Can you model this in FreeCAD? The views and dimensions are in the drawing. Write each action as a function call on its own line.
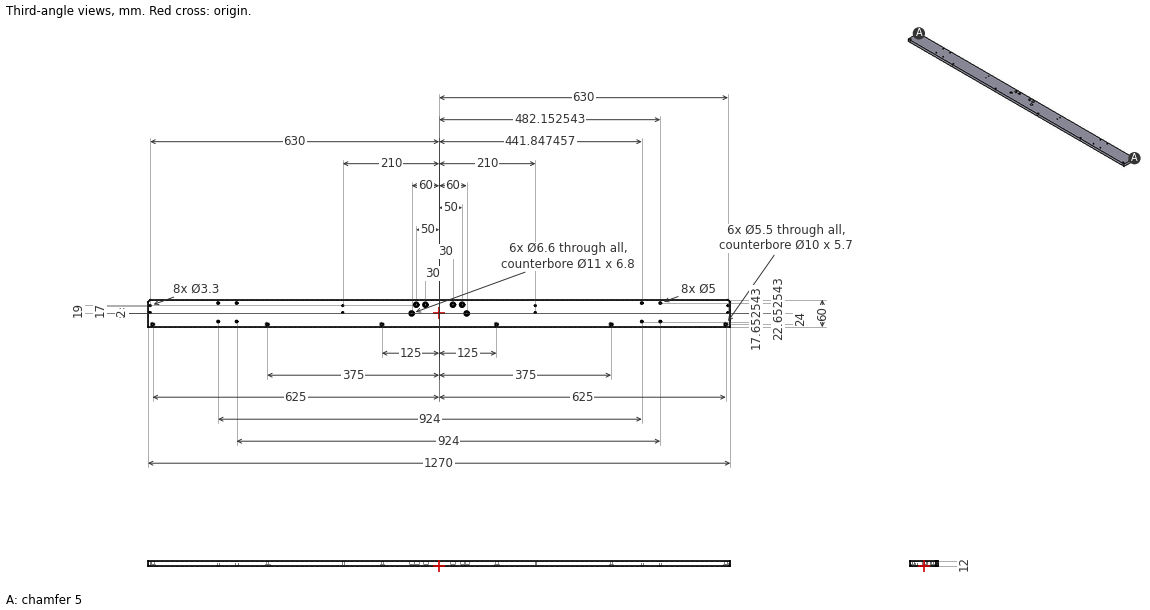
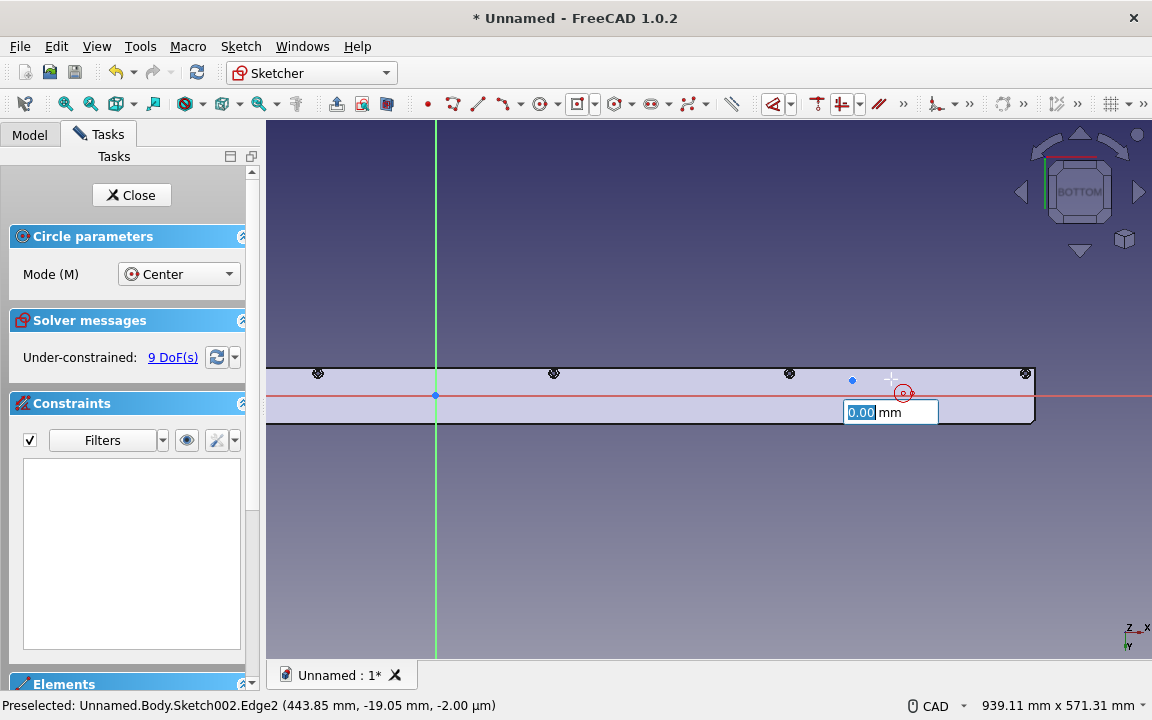
scroll(892, 378, up, 10)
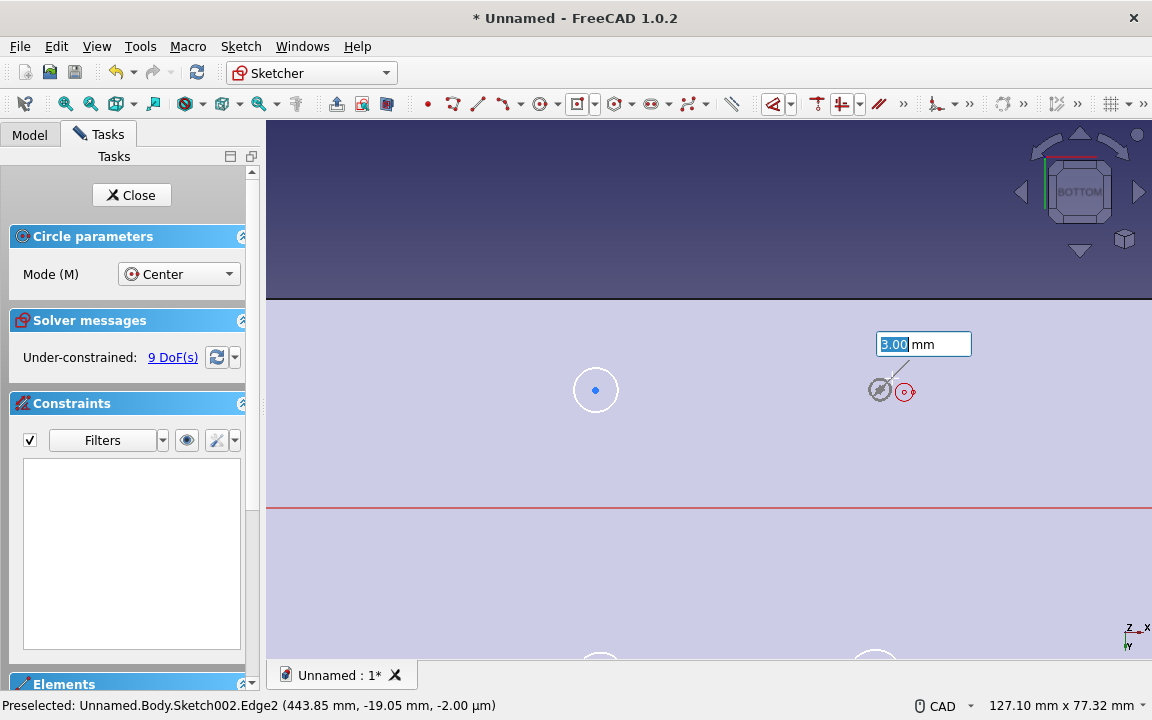
click(891, 373)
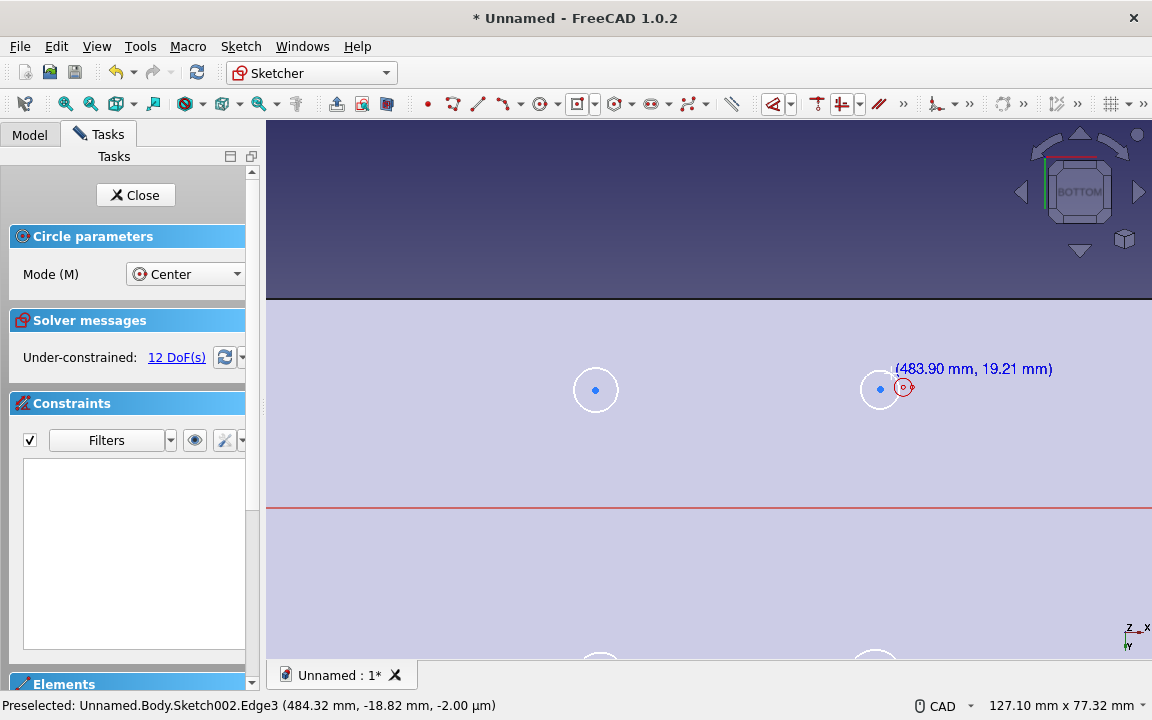
scroll(891, 379, down, 13)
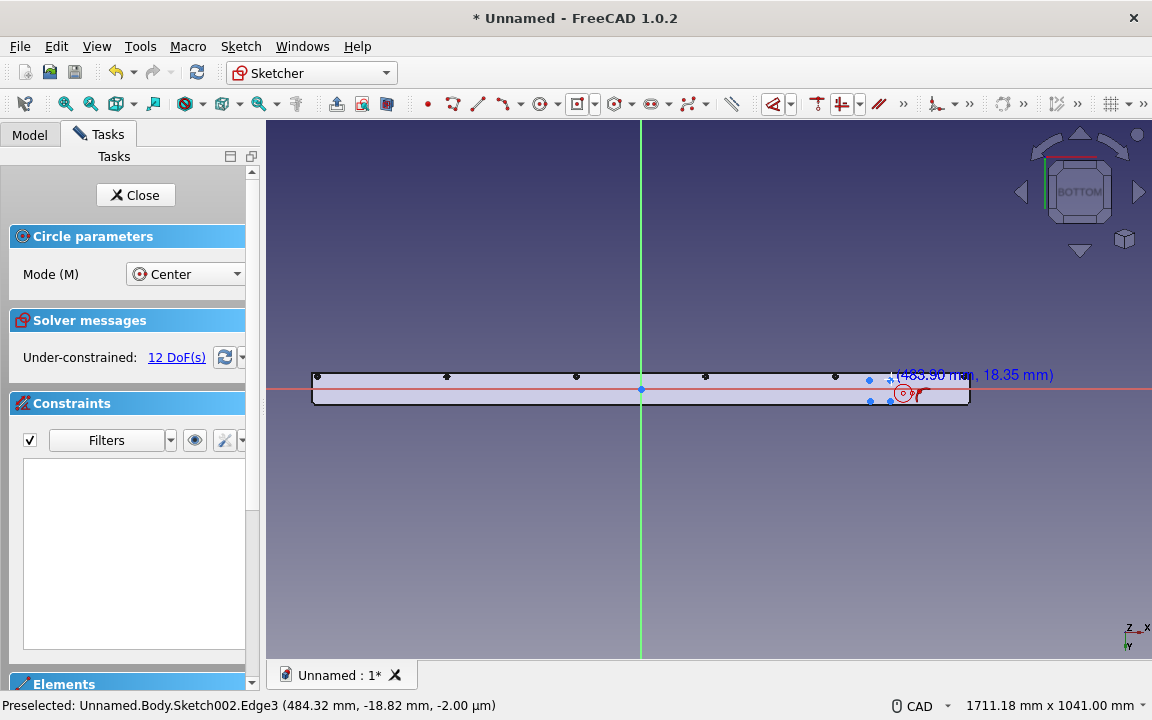
scroll(391, 380, up, 15)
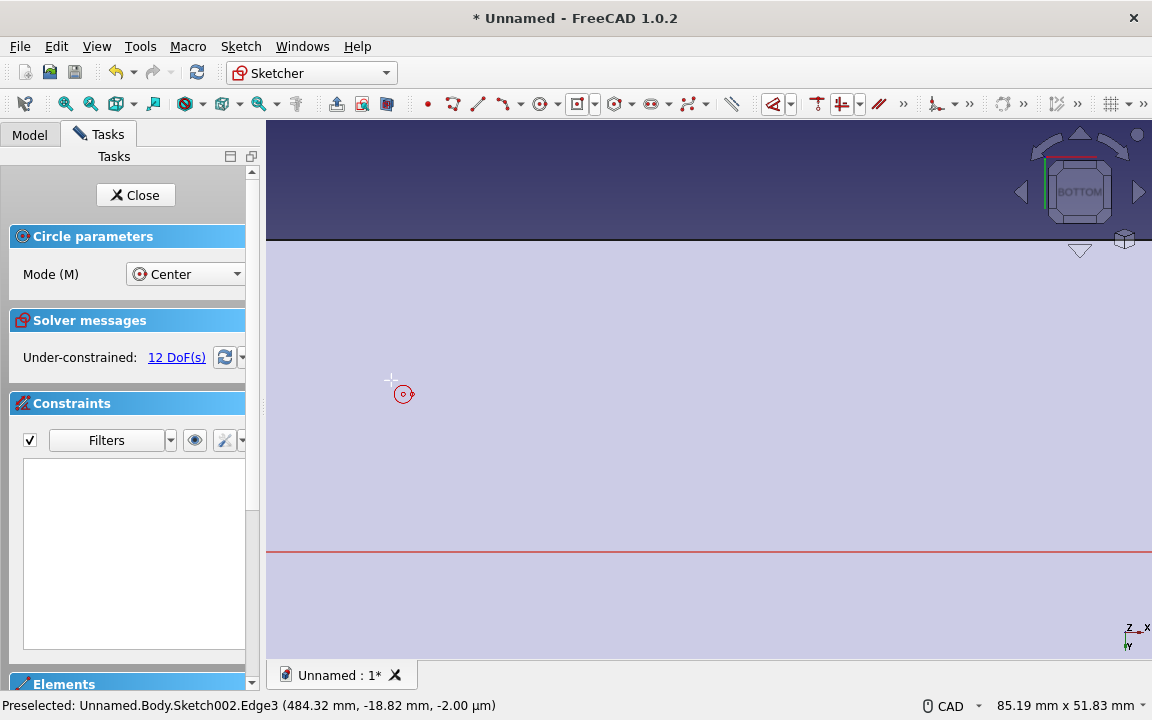
scroll(391, 380, down, 15)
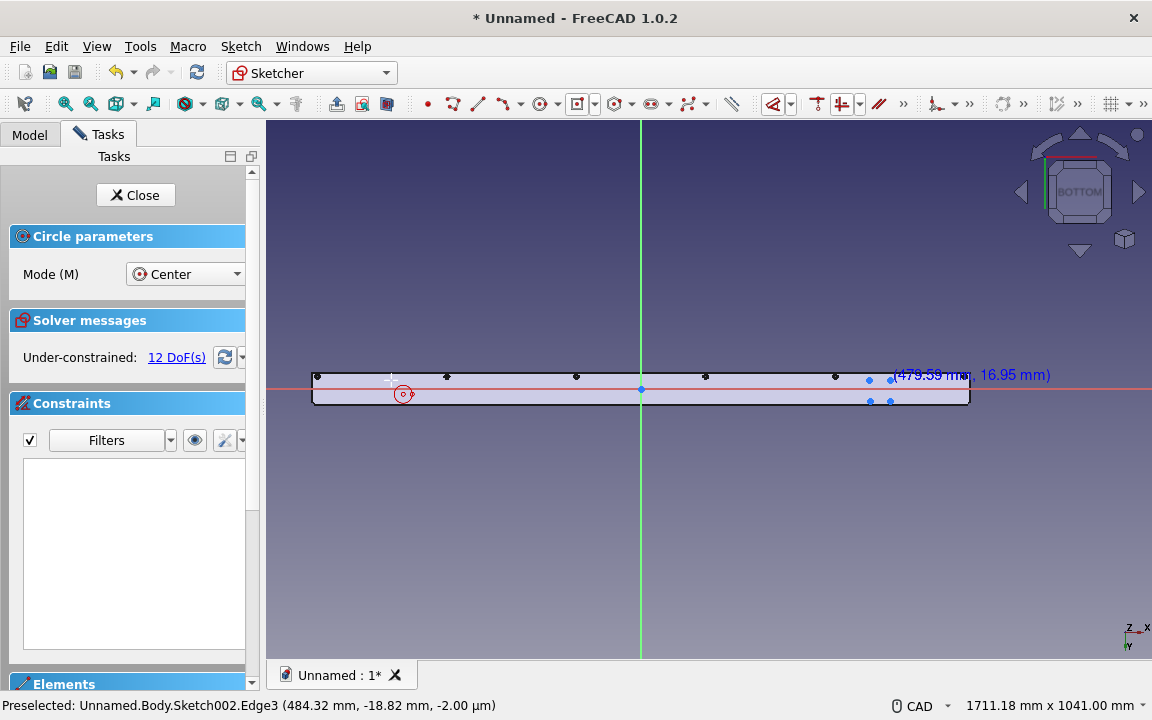
scroll(391, 380, up, 3)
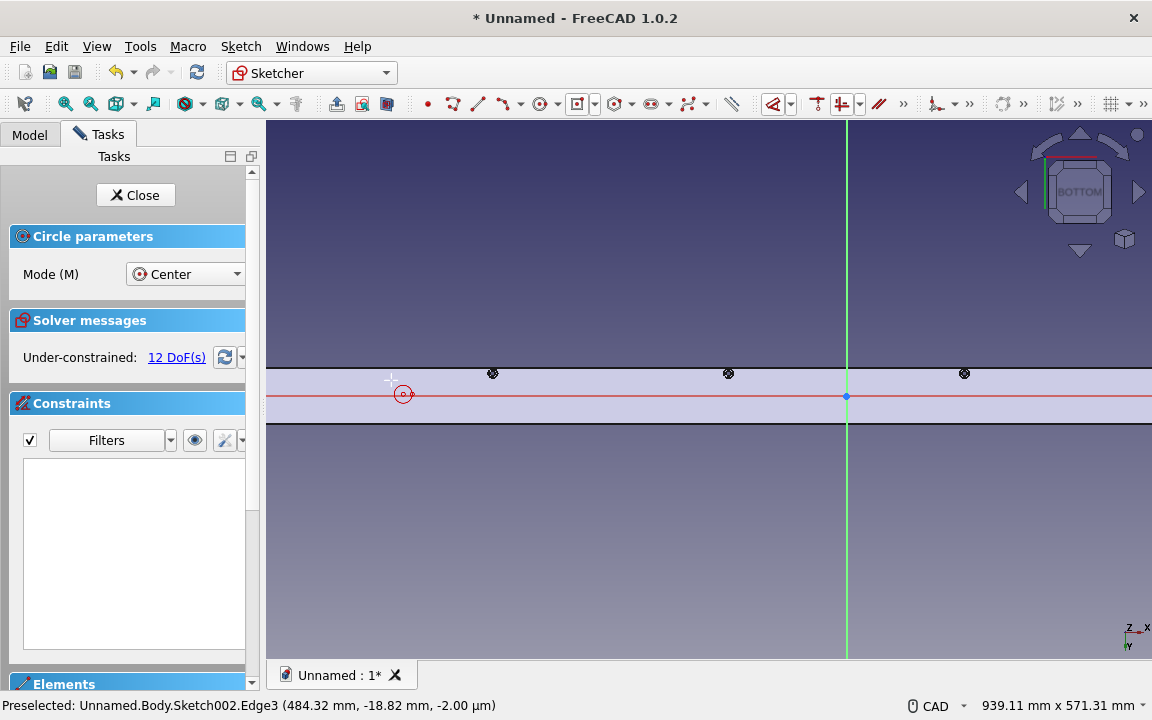
click(392, 379)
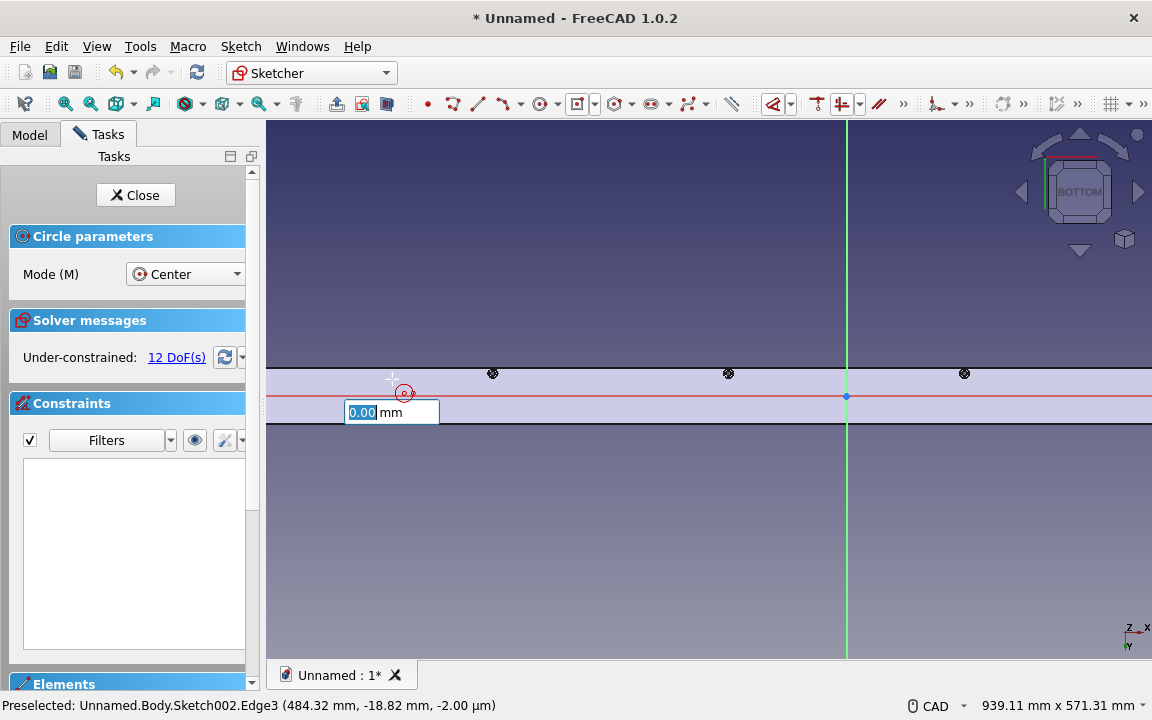
scroll(393, 378, up, 10)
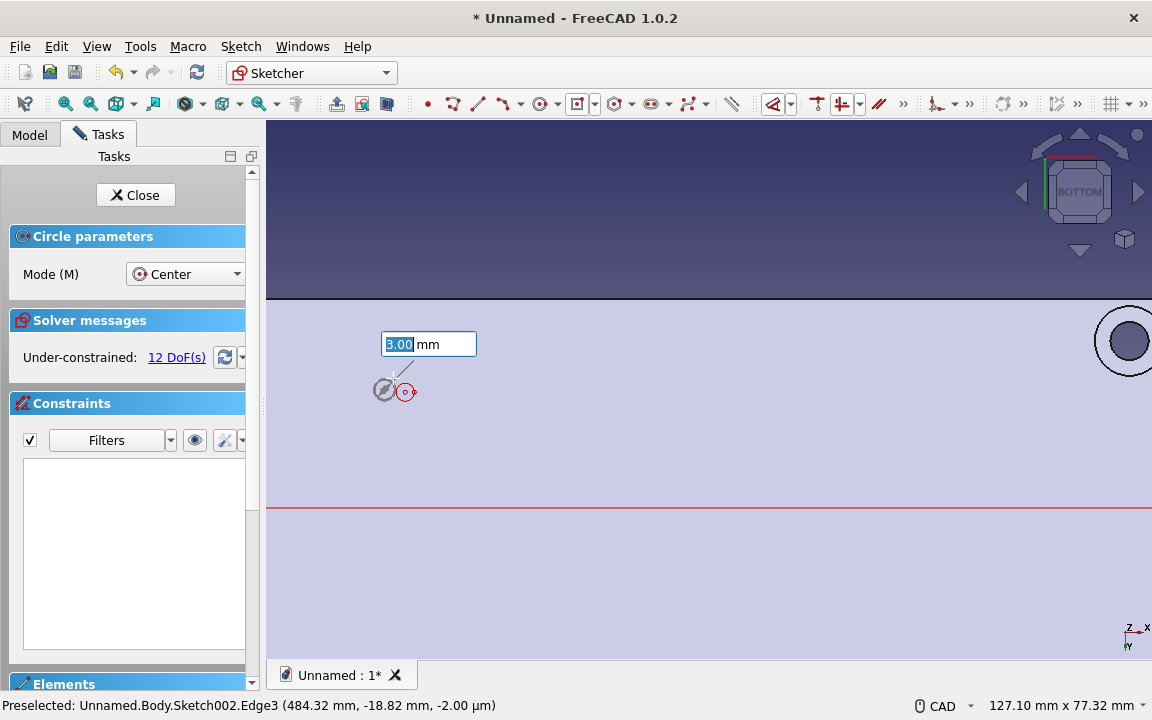
click(395, 373)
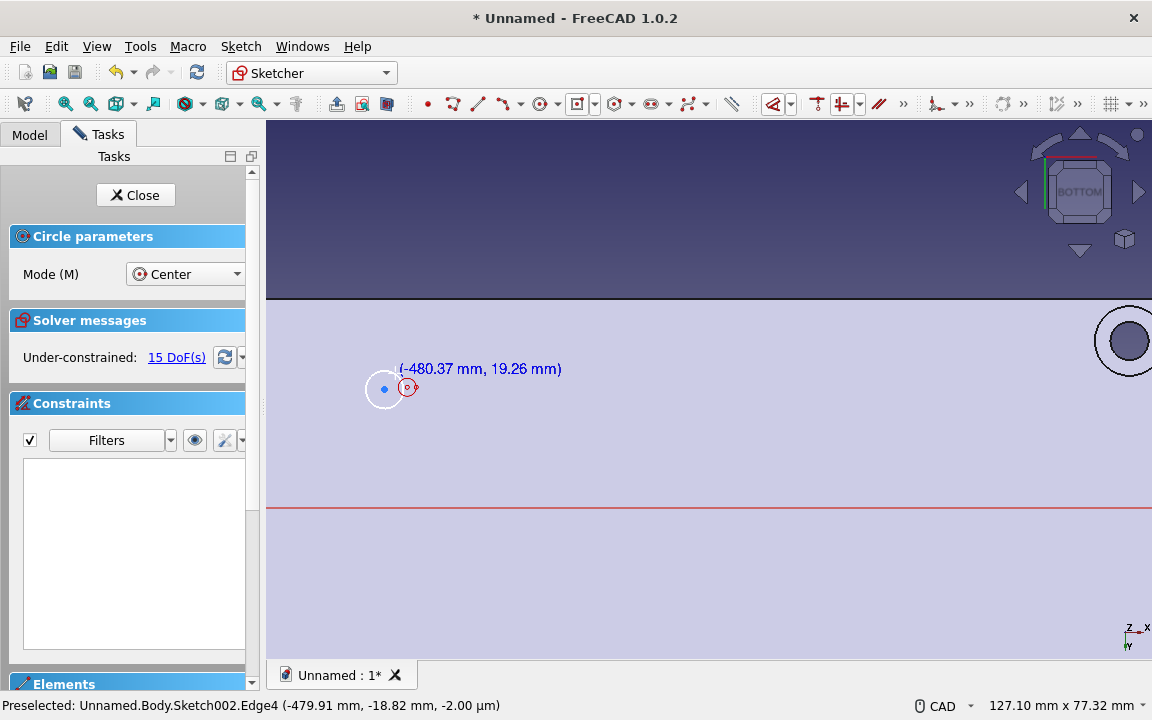
scroll(664, 385, up, 2)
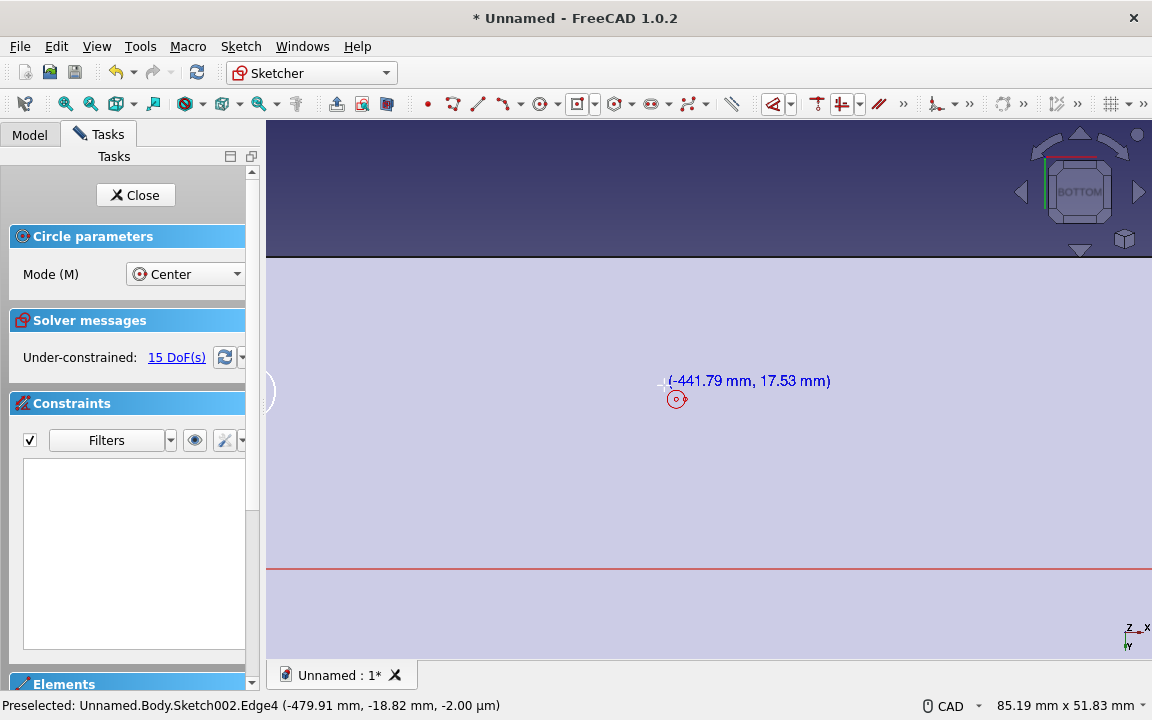
scroll(399, 379, down, 15)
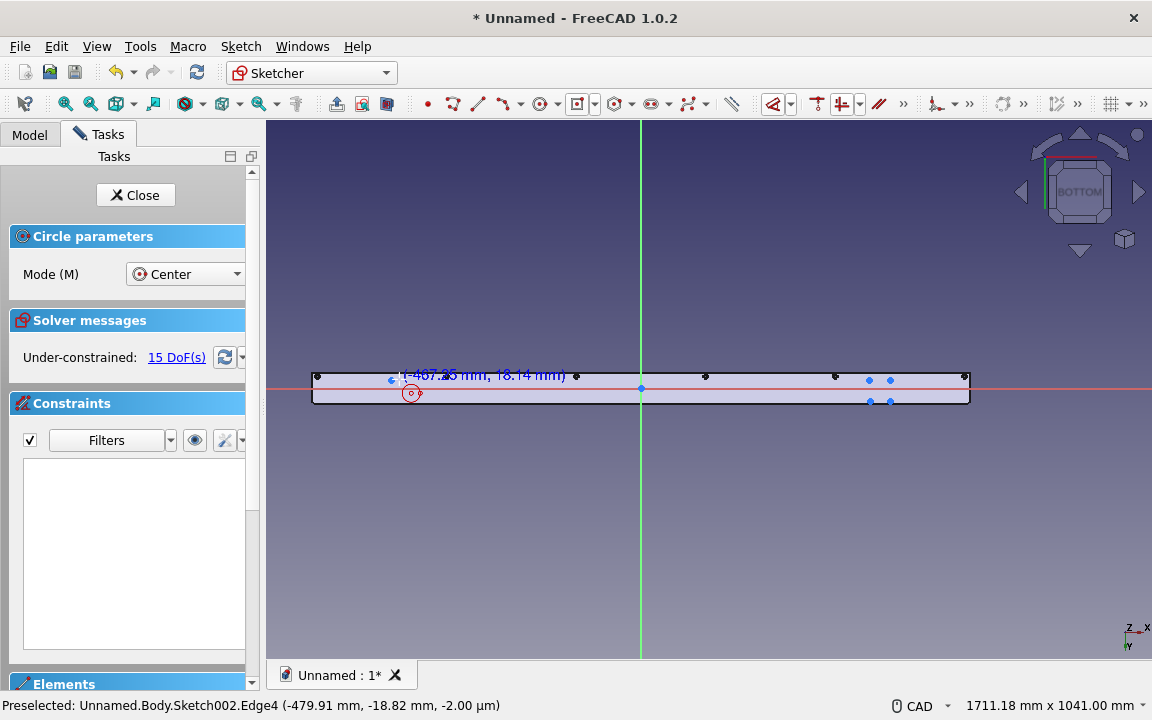
scroll(412, 380, up, 3)